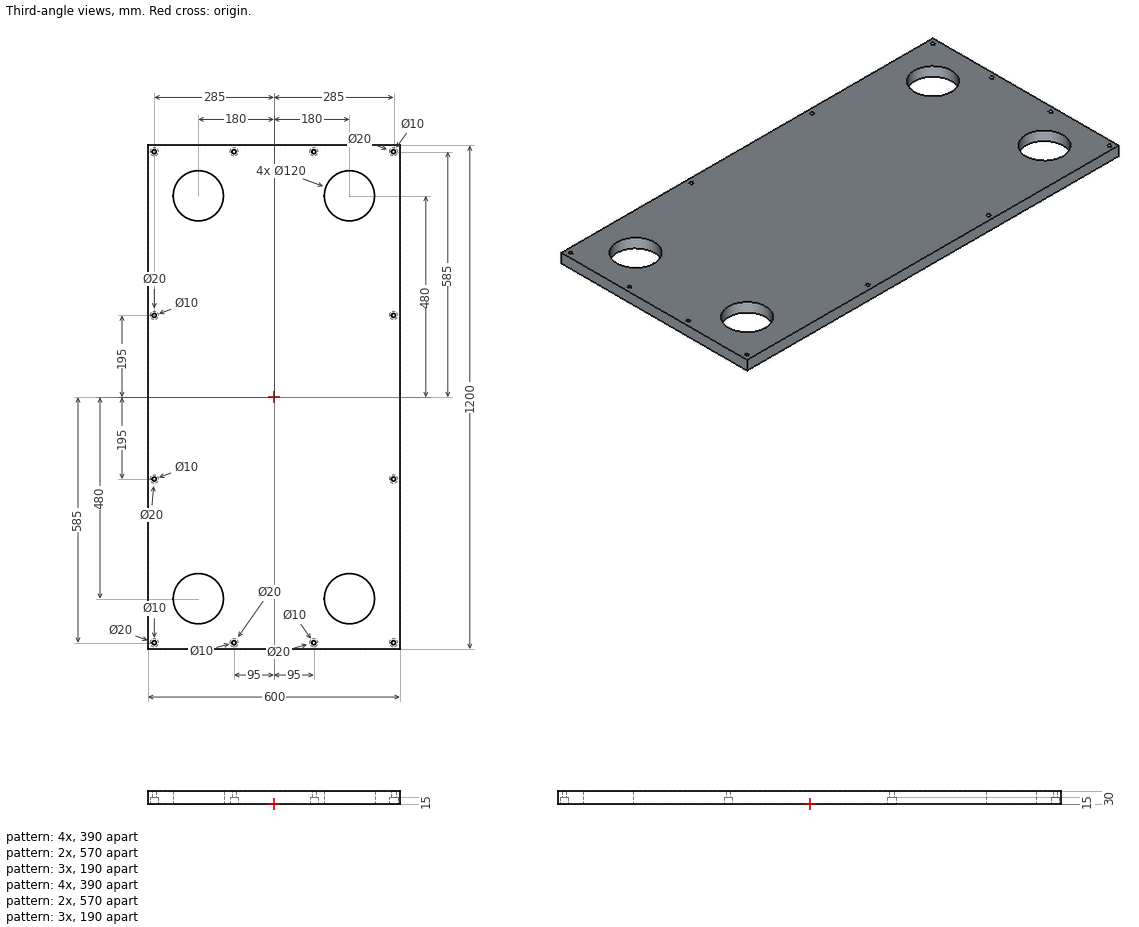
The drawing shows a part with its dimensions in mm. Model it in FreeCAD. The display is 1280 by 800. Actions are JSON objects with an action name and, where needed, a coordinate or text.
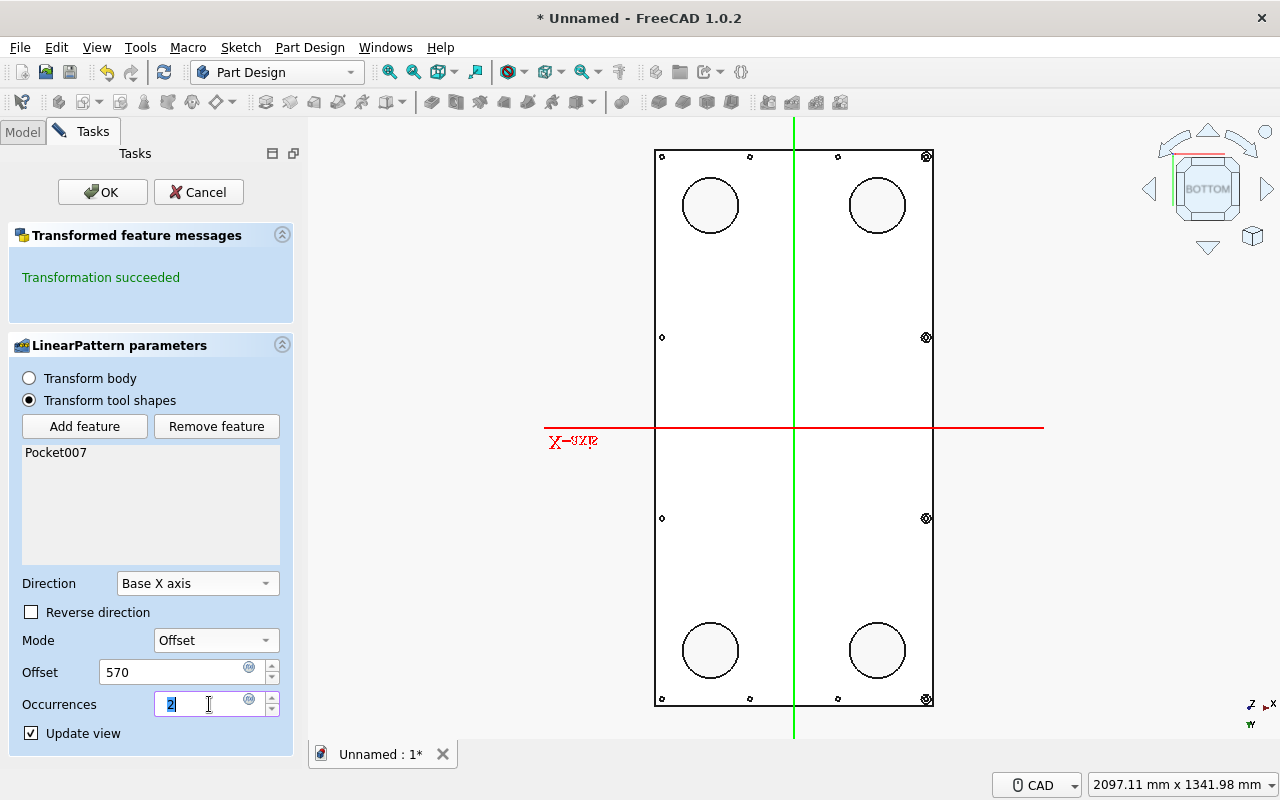
{"action": "type", "text": "2"}
{"action": "key", "text": "Tab"}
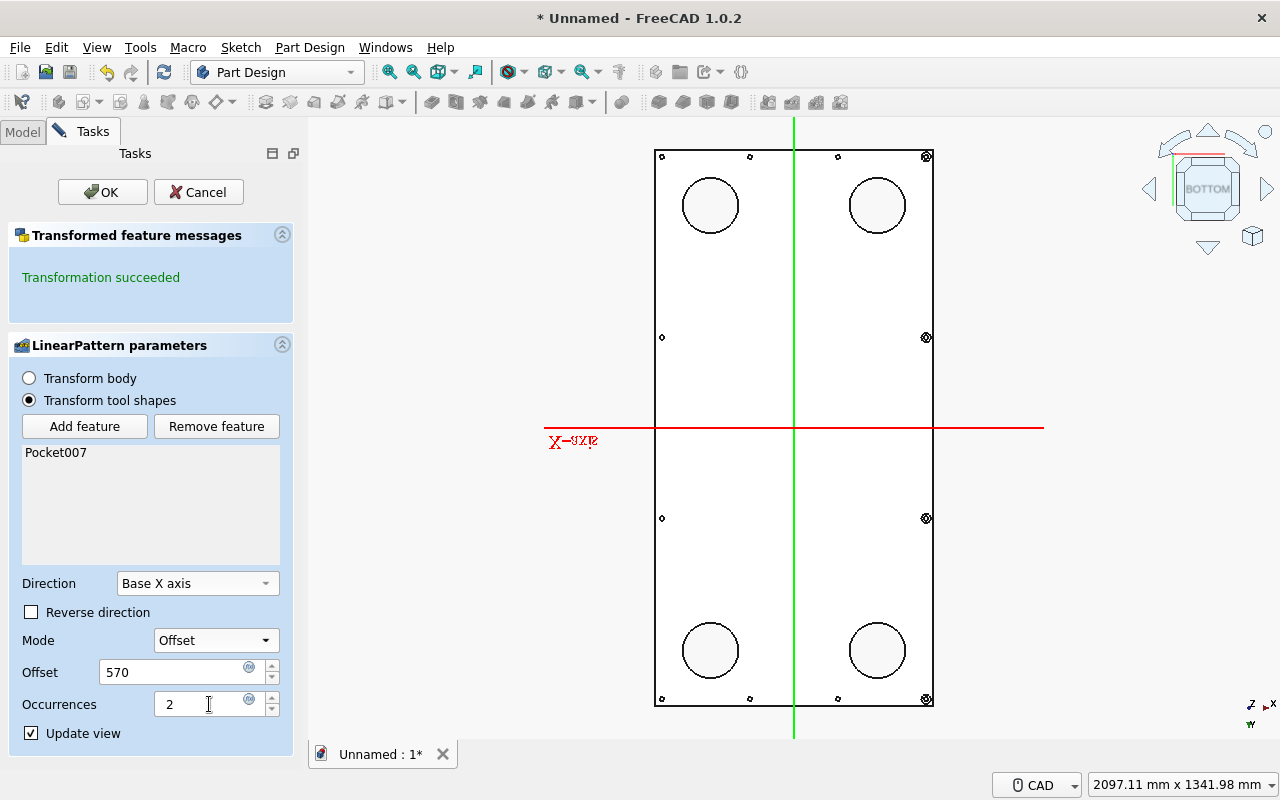
{"action": "left_click", "coordinate": [30, 612]}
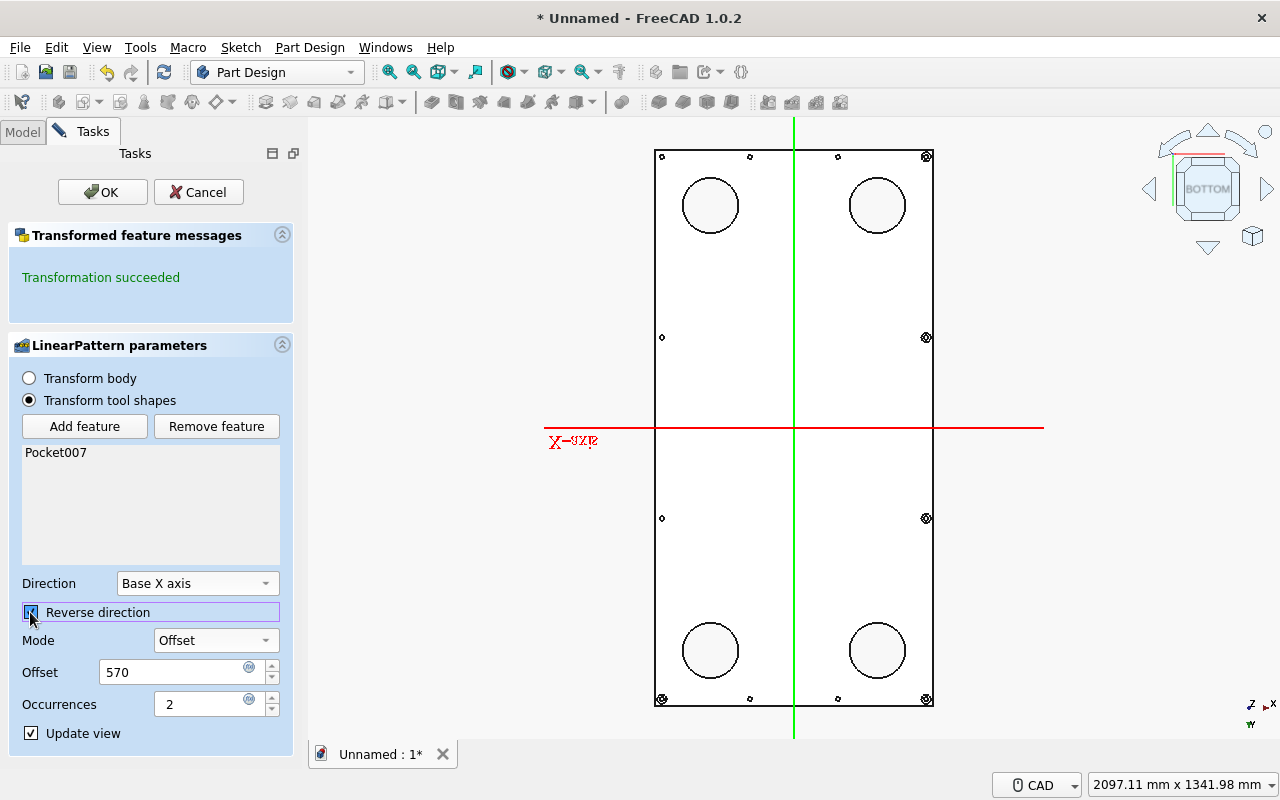
{"action": "left_click", "coordinate": [103, 192]}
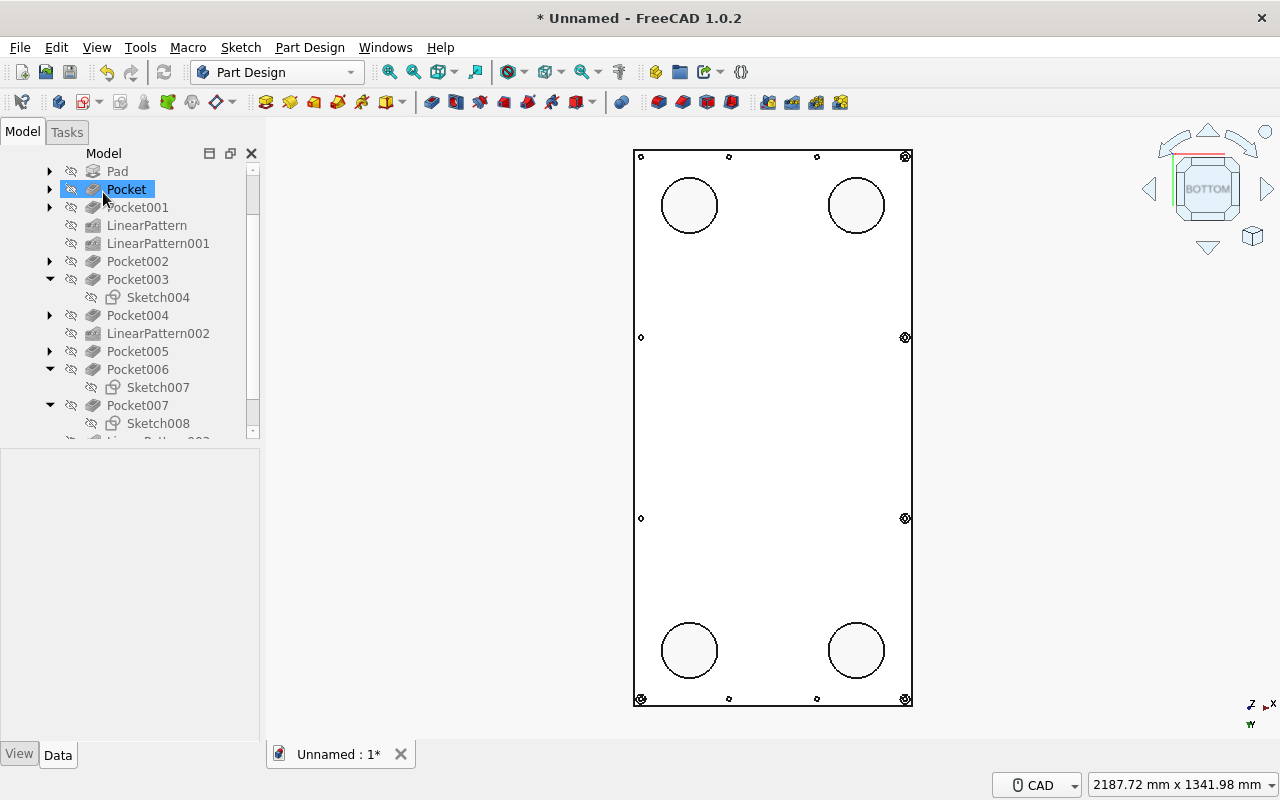
{"action": "left_click", "coordinate": [84, 102]}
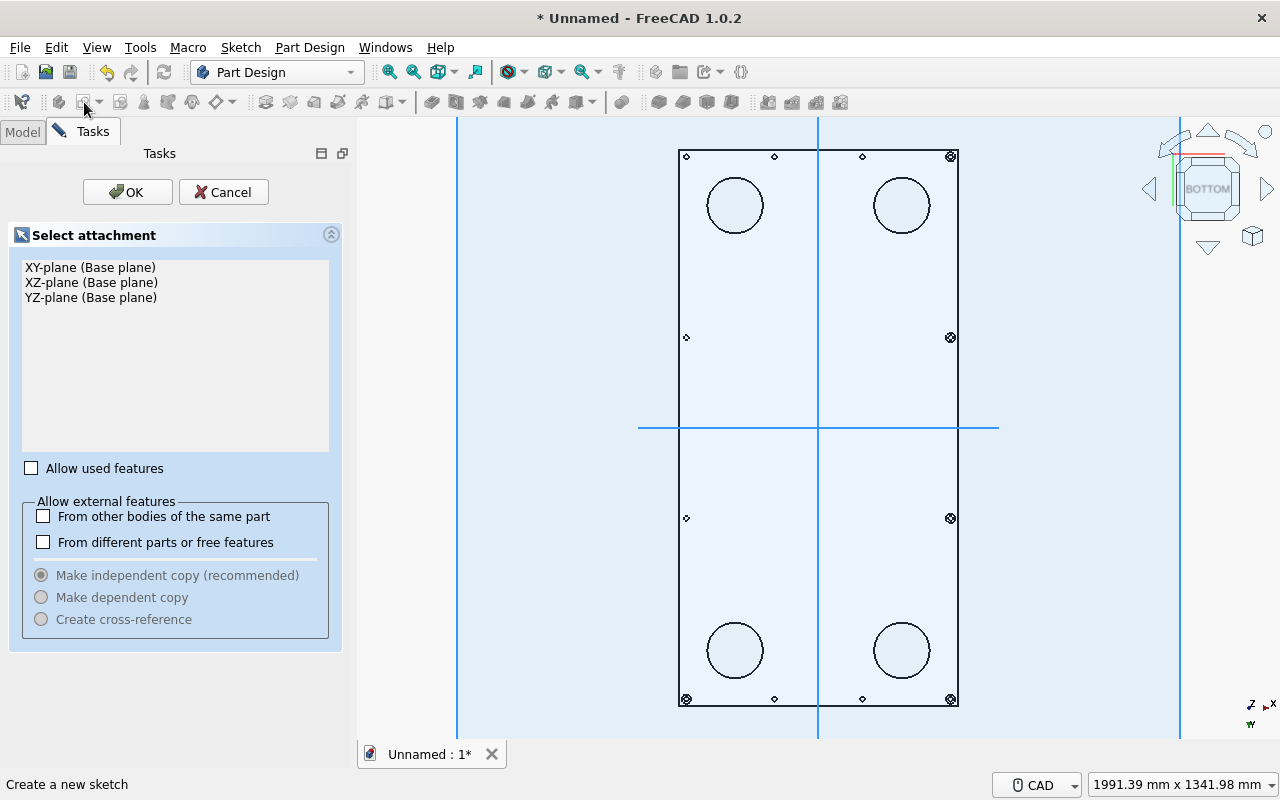
{"action": "left_click", "coordinate": [82, 268]}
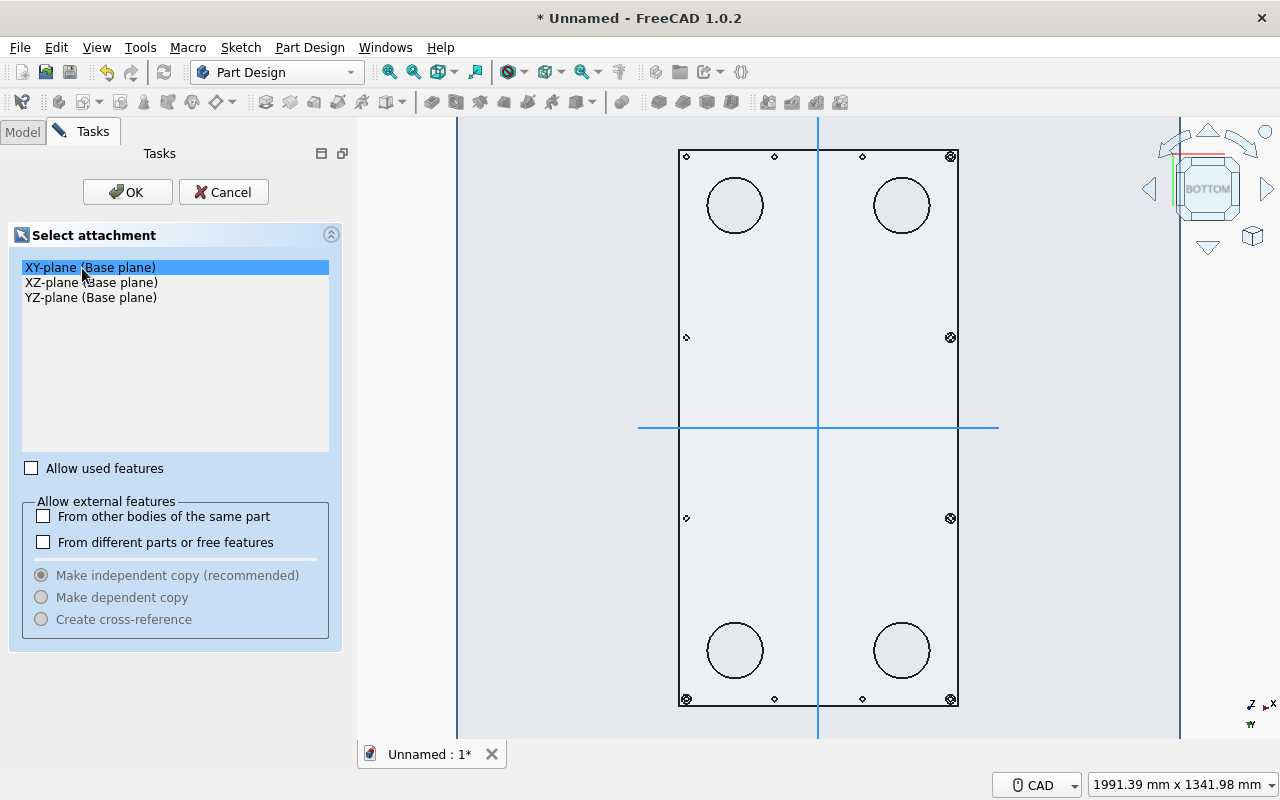
{"action": "left_click", "coordinate": [128, 192]}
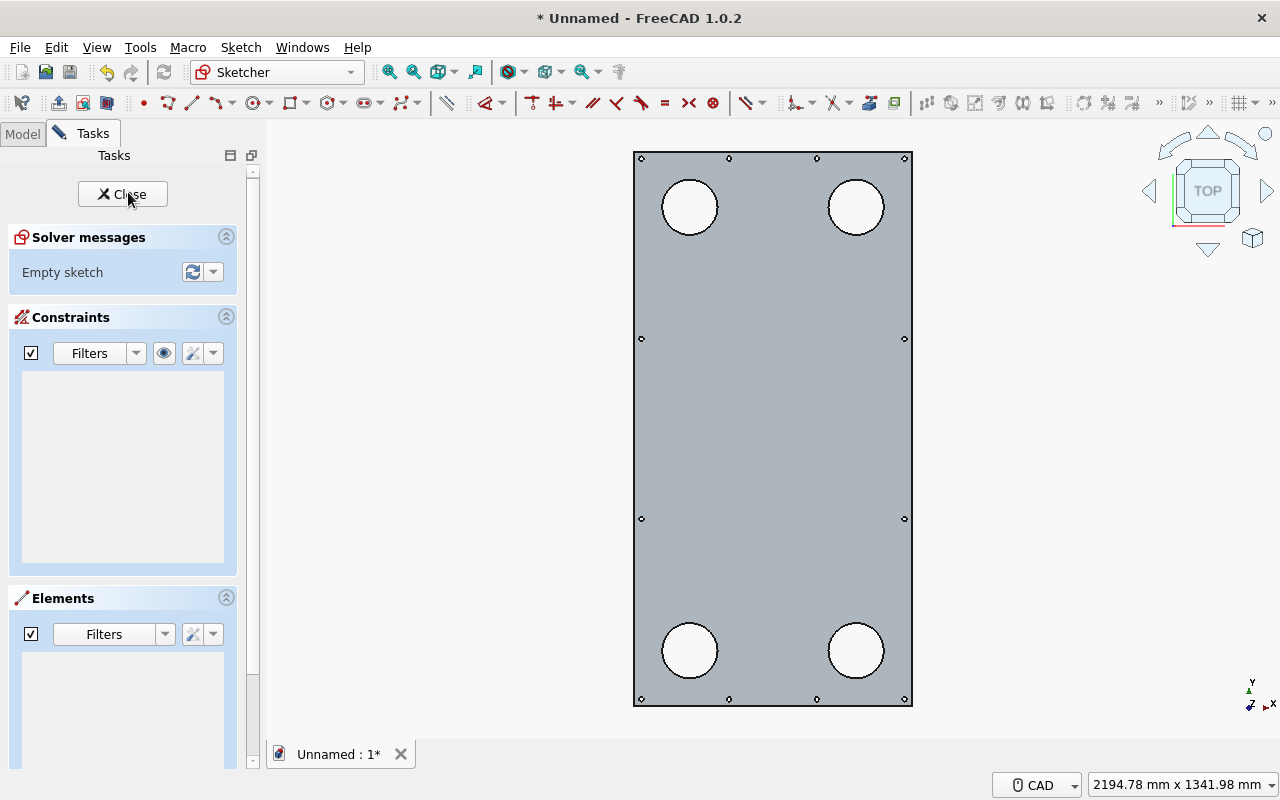
{"action": "left_click", "coordinate": [108, 104]}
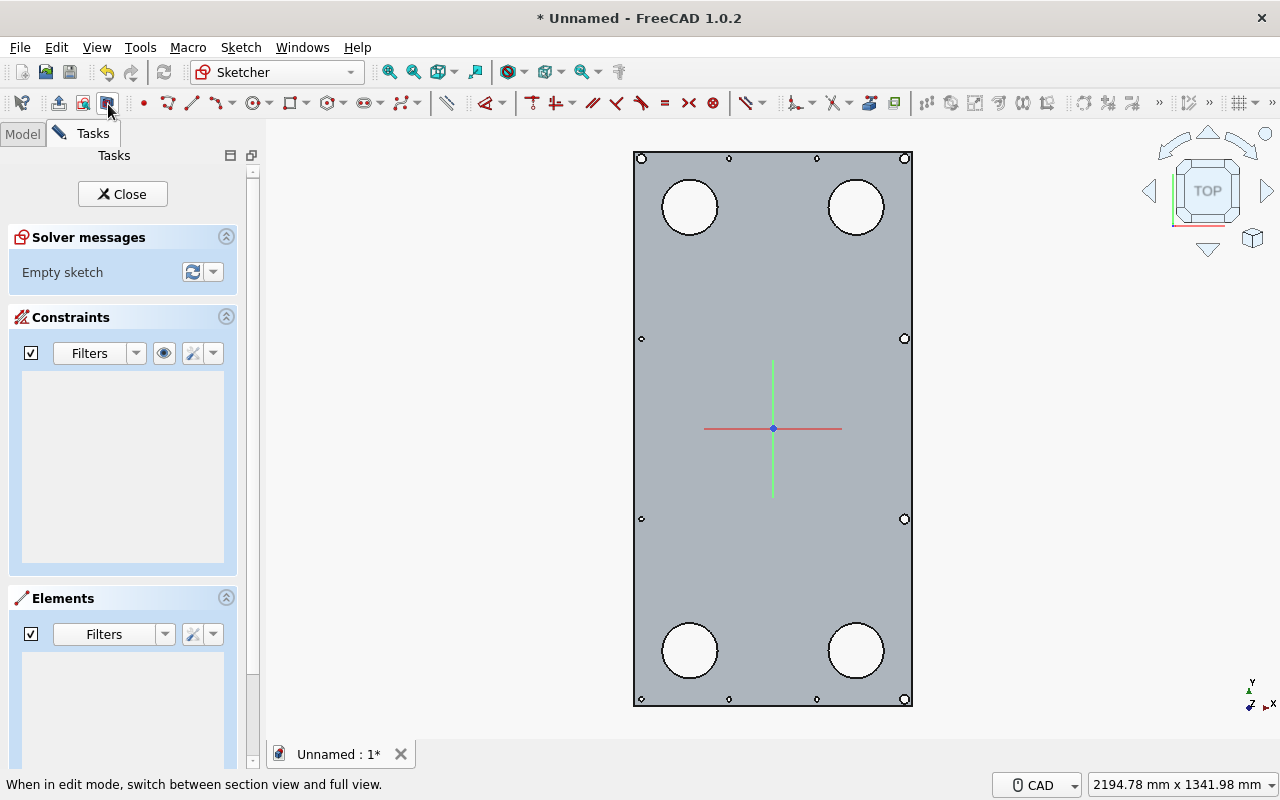
{"action": "scroll", "coordinate": [638, 334], "scroll_direction": "up", "scroll_amount": 15}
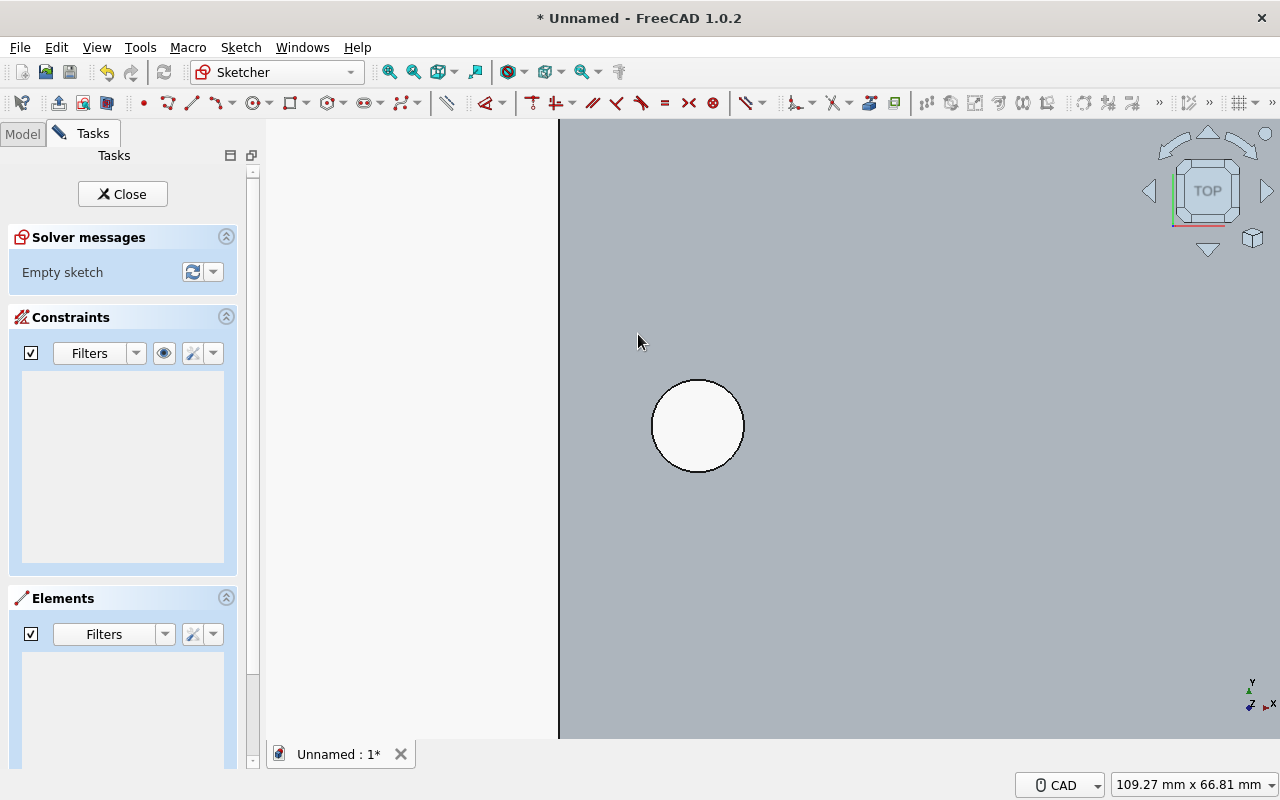
{"action": "scroll", "coordinate": [692, 423], "scroll_direction": "up", "scroll_amount": 4}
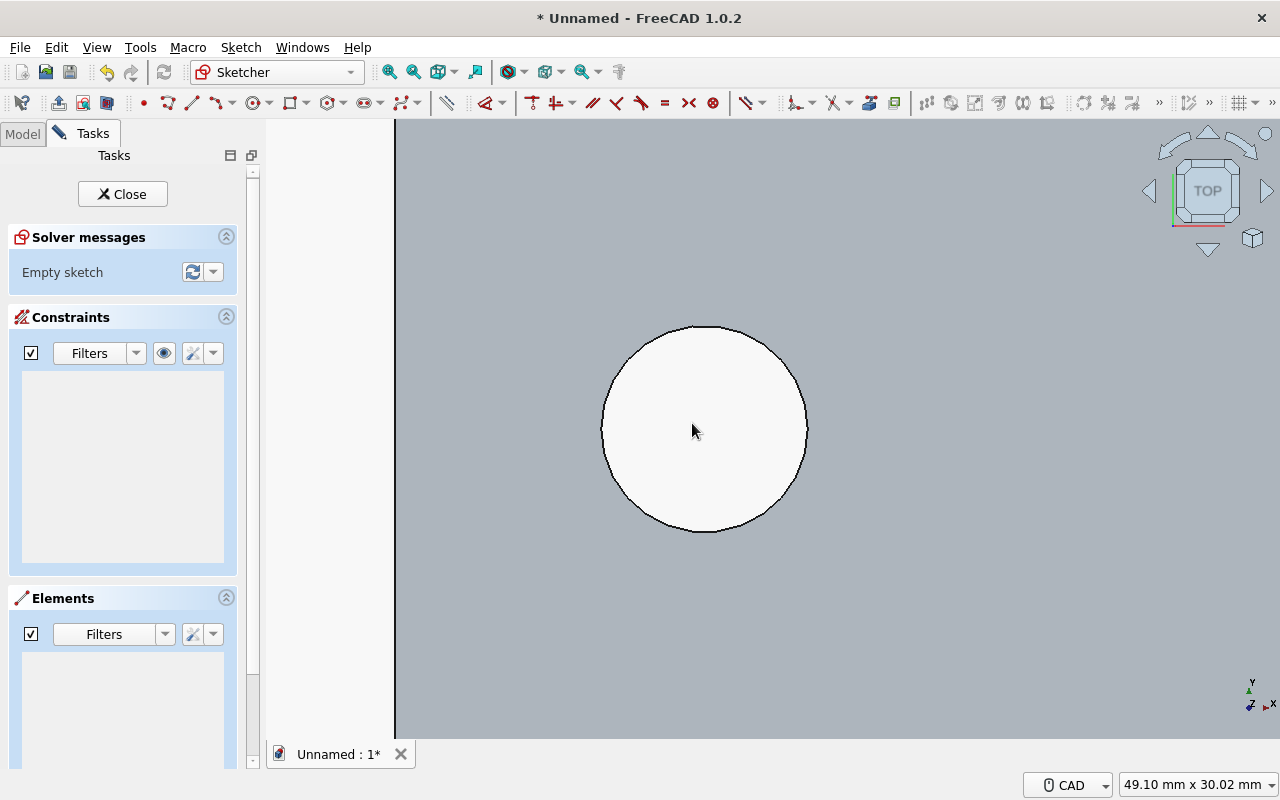
{"action": "left_click", "coordinate": [254, 104]}